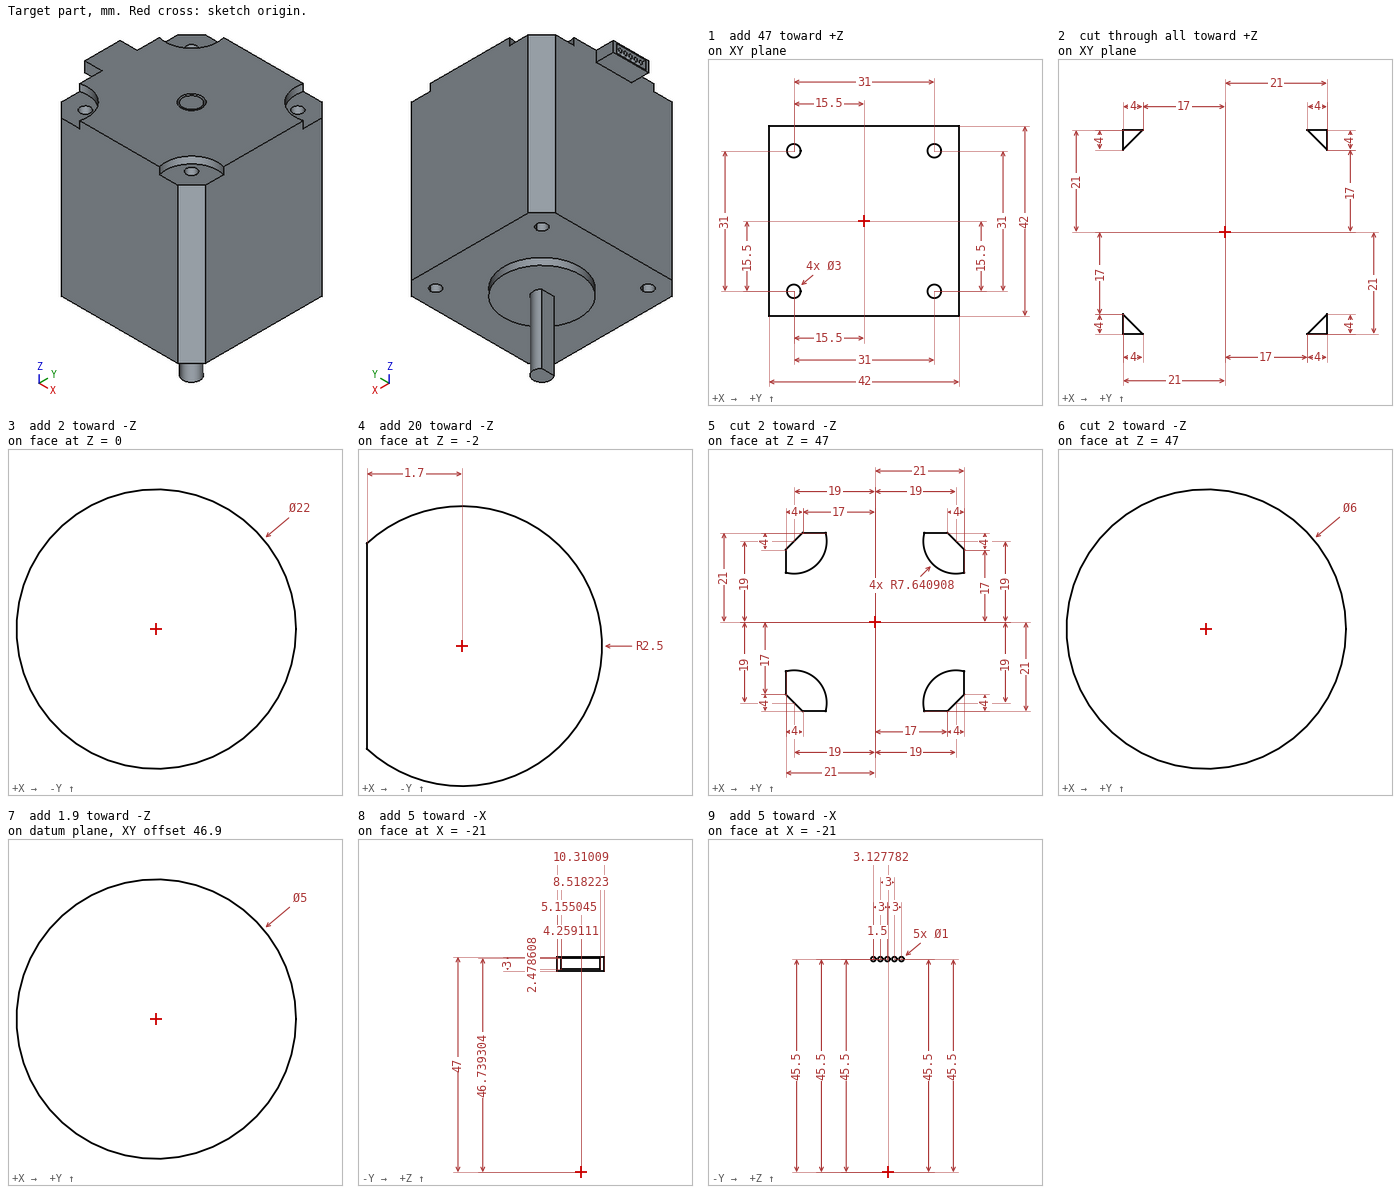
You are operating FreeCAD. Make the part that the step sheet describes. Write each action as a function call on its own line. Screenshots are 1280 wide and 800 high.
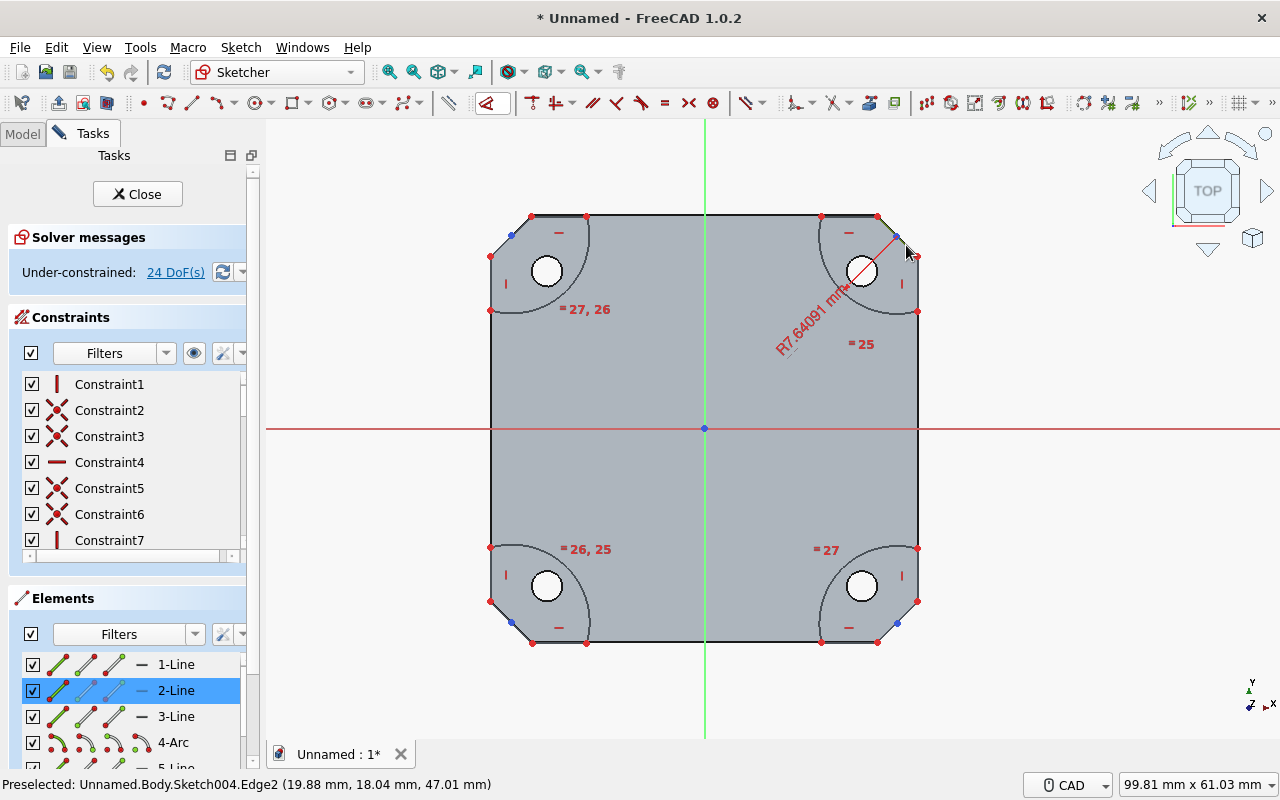
key(l)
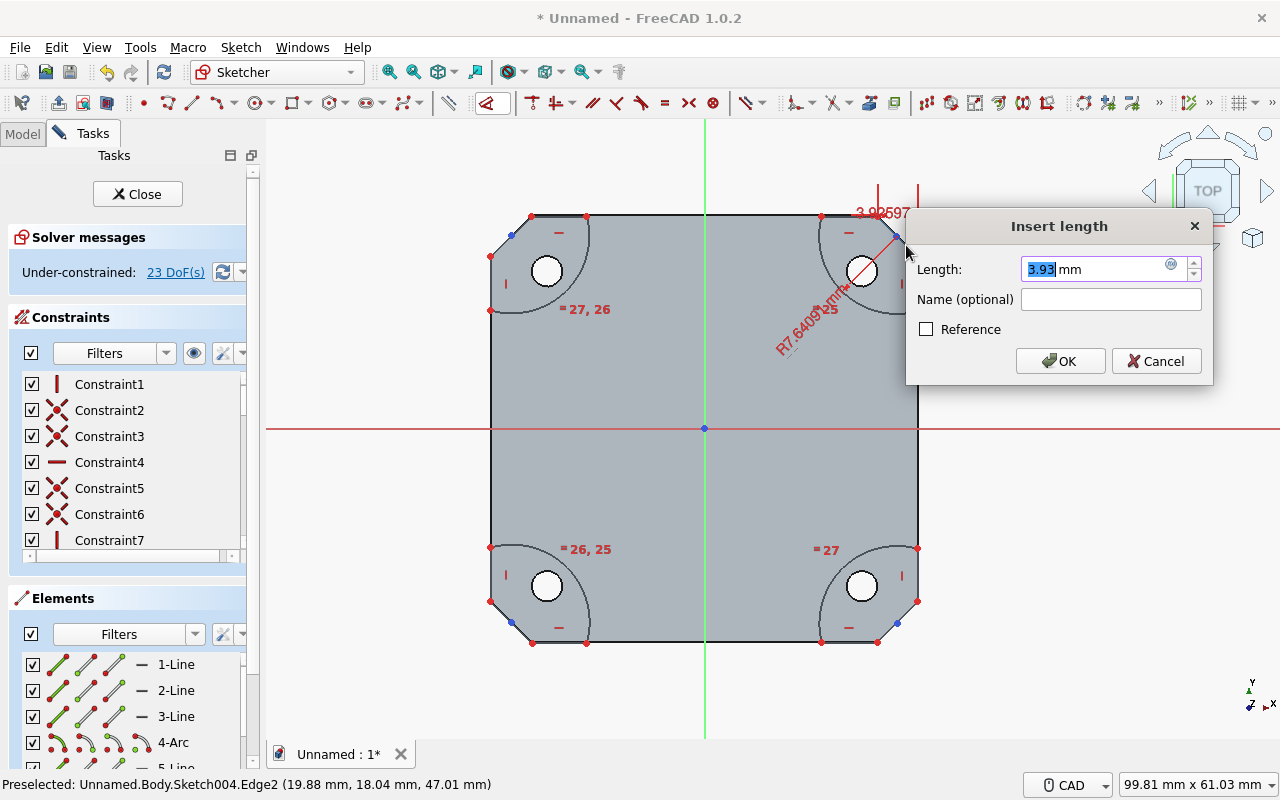
text(4)
key(Return)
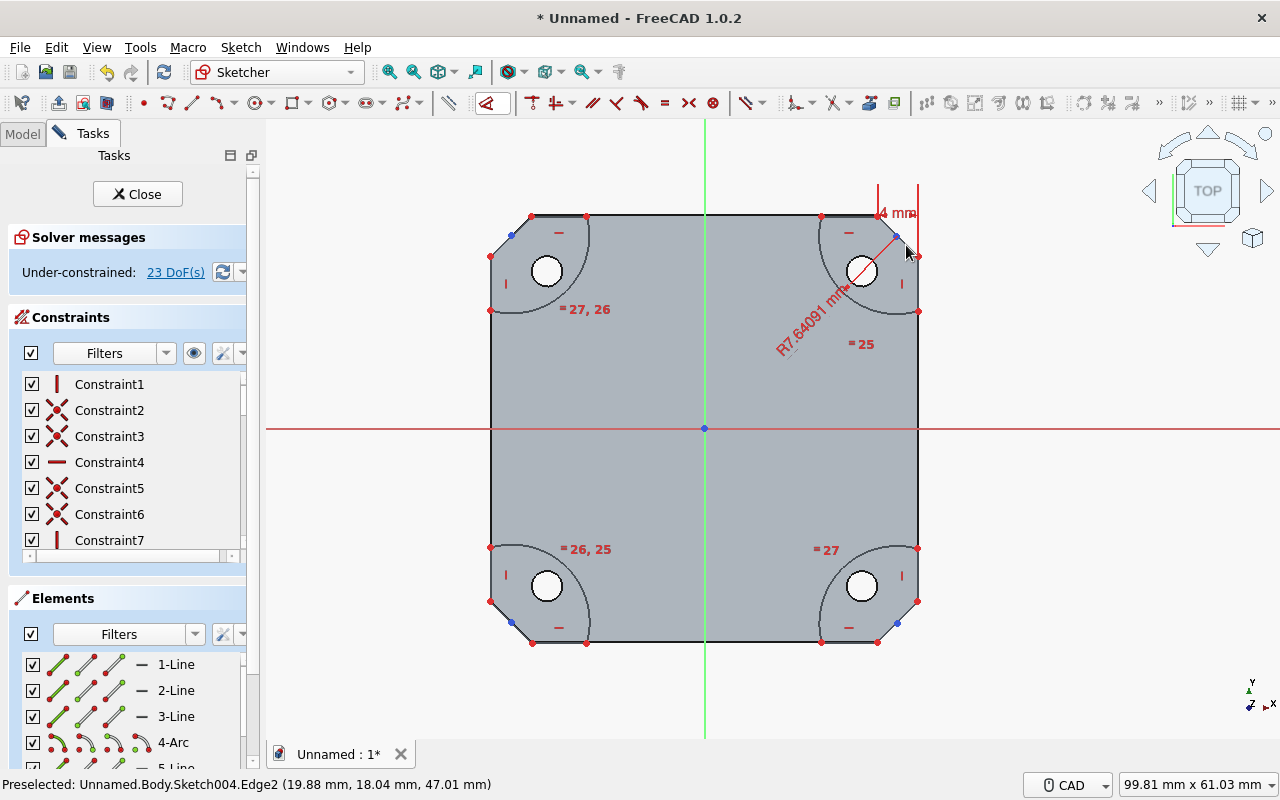
click(906, 245)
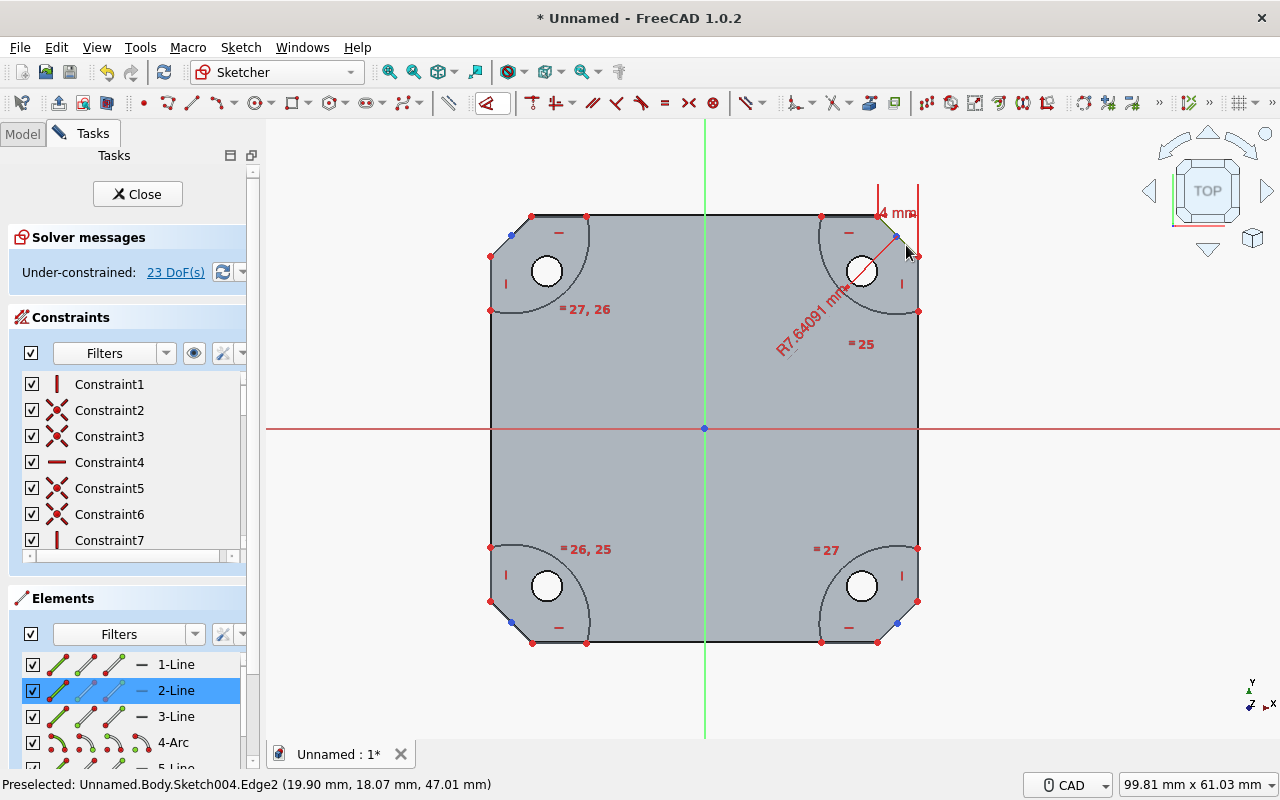
key(i)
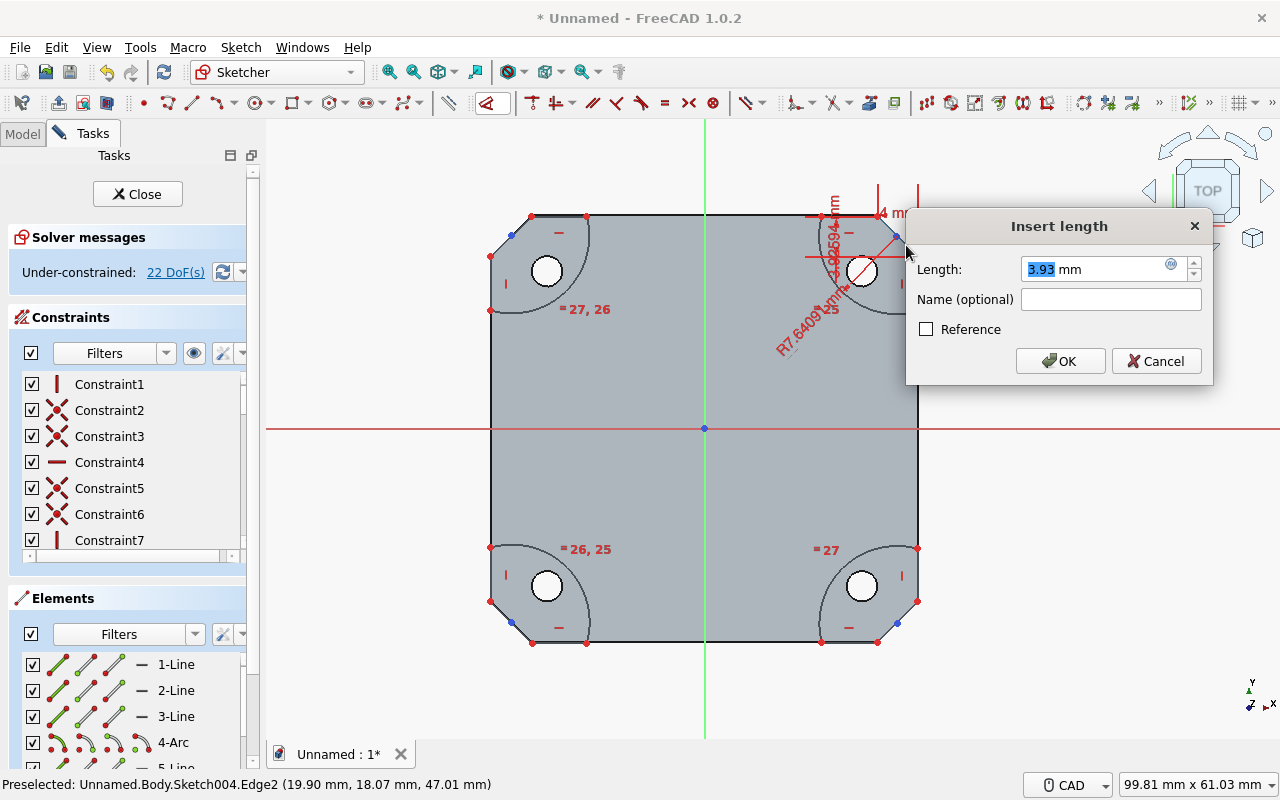
text(4)
key(Return)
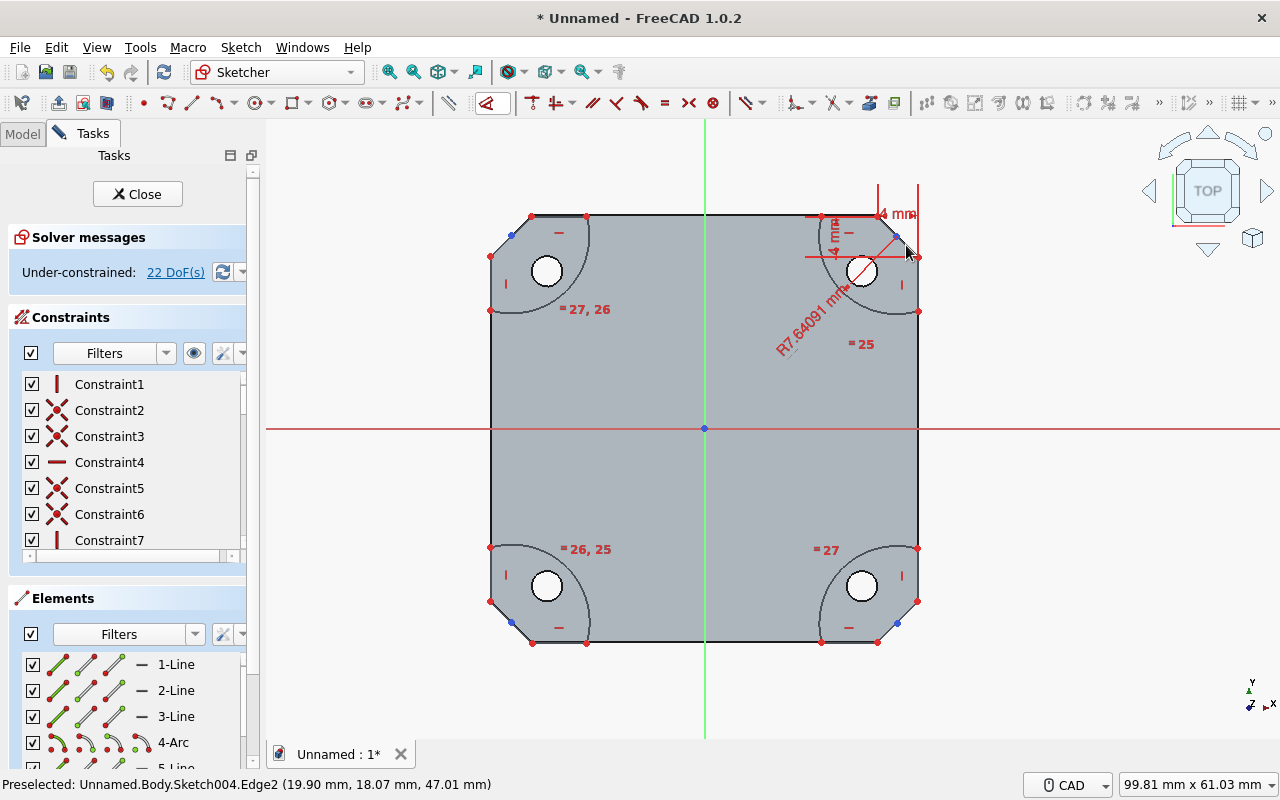
click(503, 614)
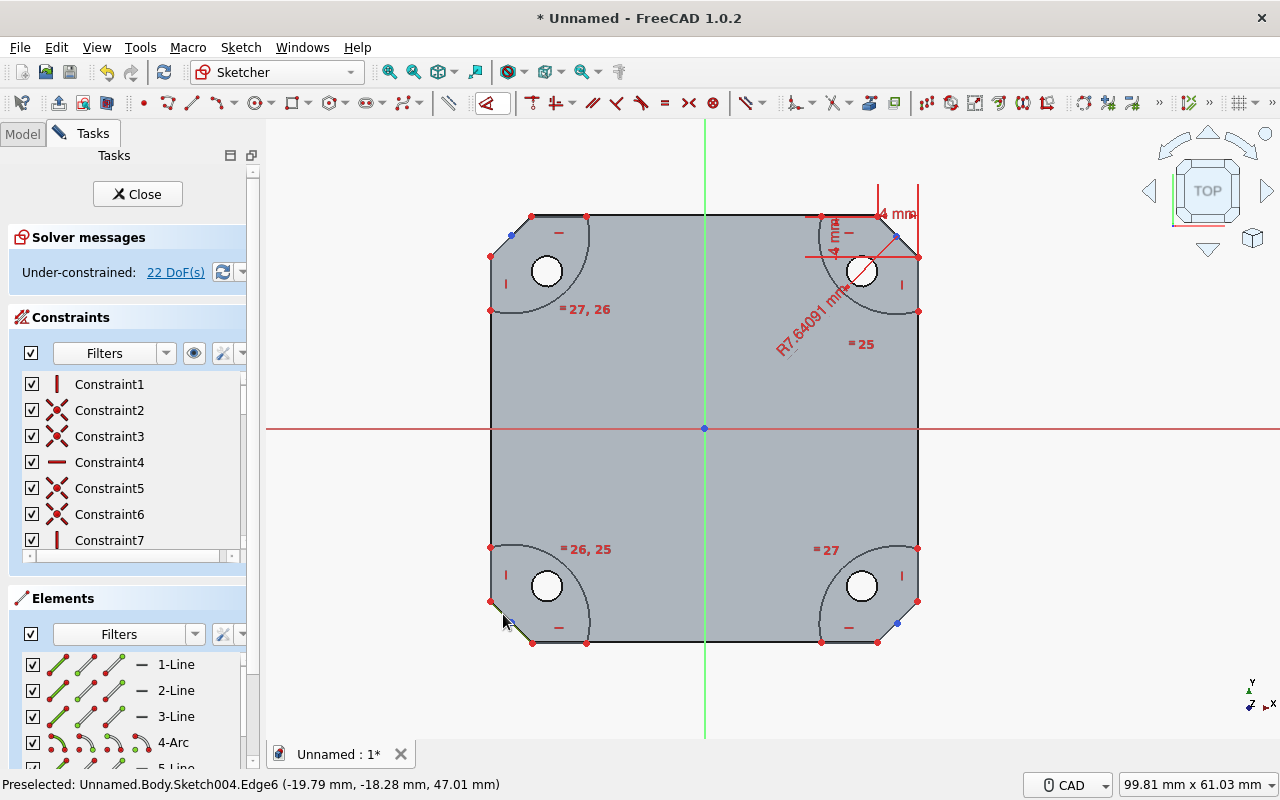
click(504, 104)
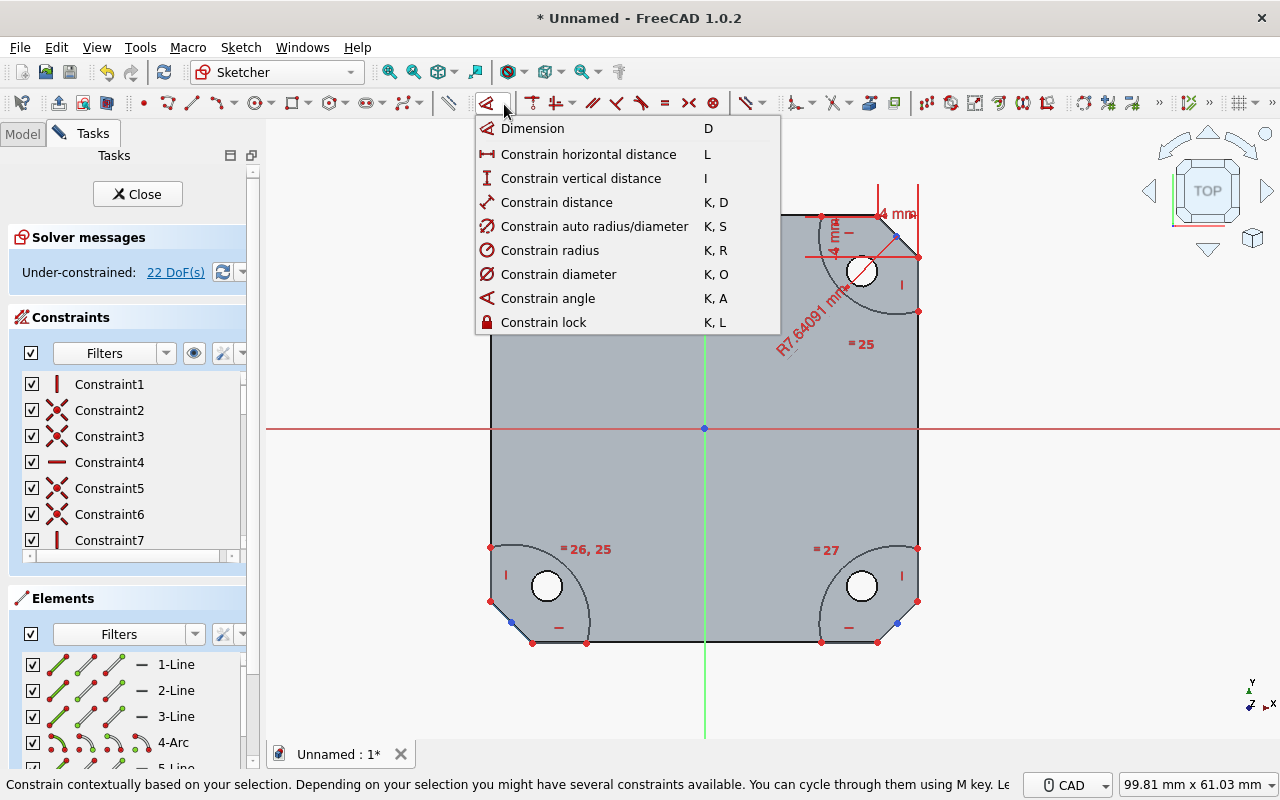
click(628, 154)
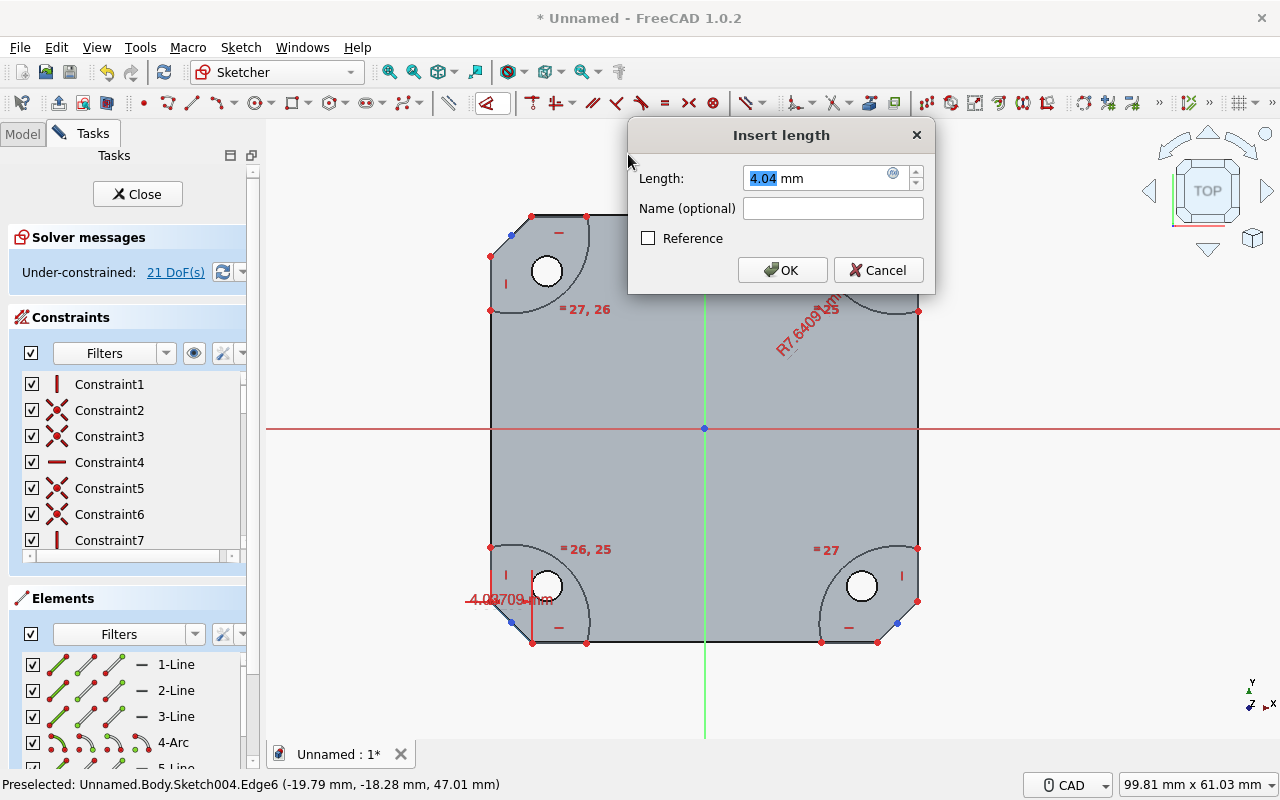
text(4)
key(Return)